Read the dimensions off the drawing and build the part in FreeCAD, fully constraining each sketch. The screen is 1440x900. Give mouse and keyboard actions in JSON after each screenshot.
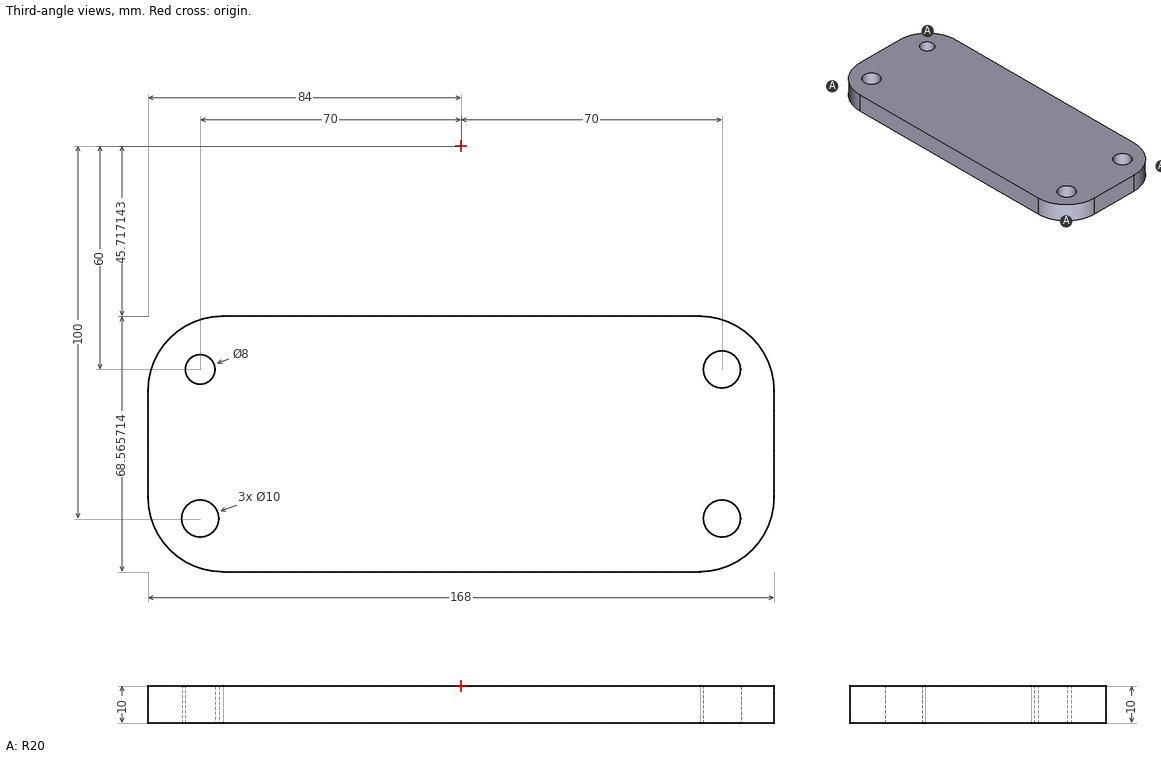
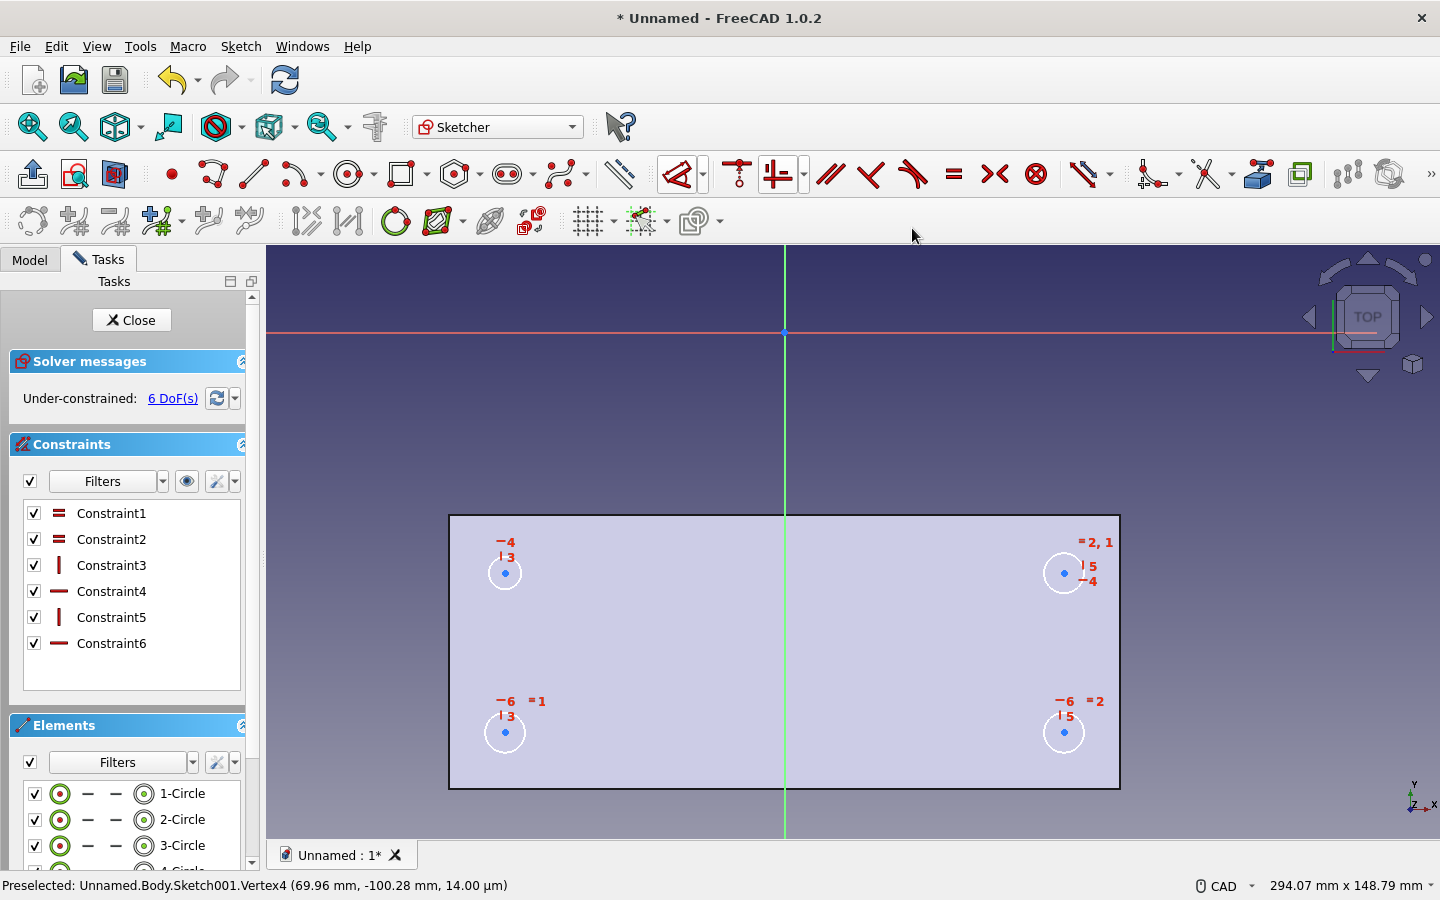
{"action": "scroll", "coordinate": [516, 562], "scroll_direction": "up", "scroll_amount": 2}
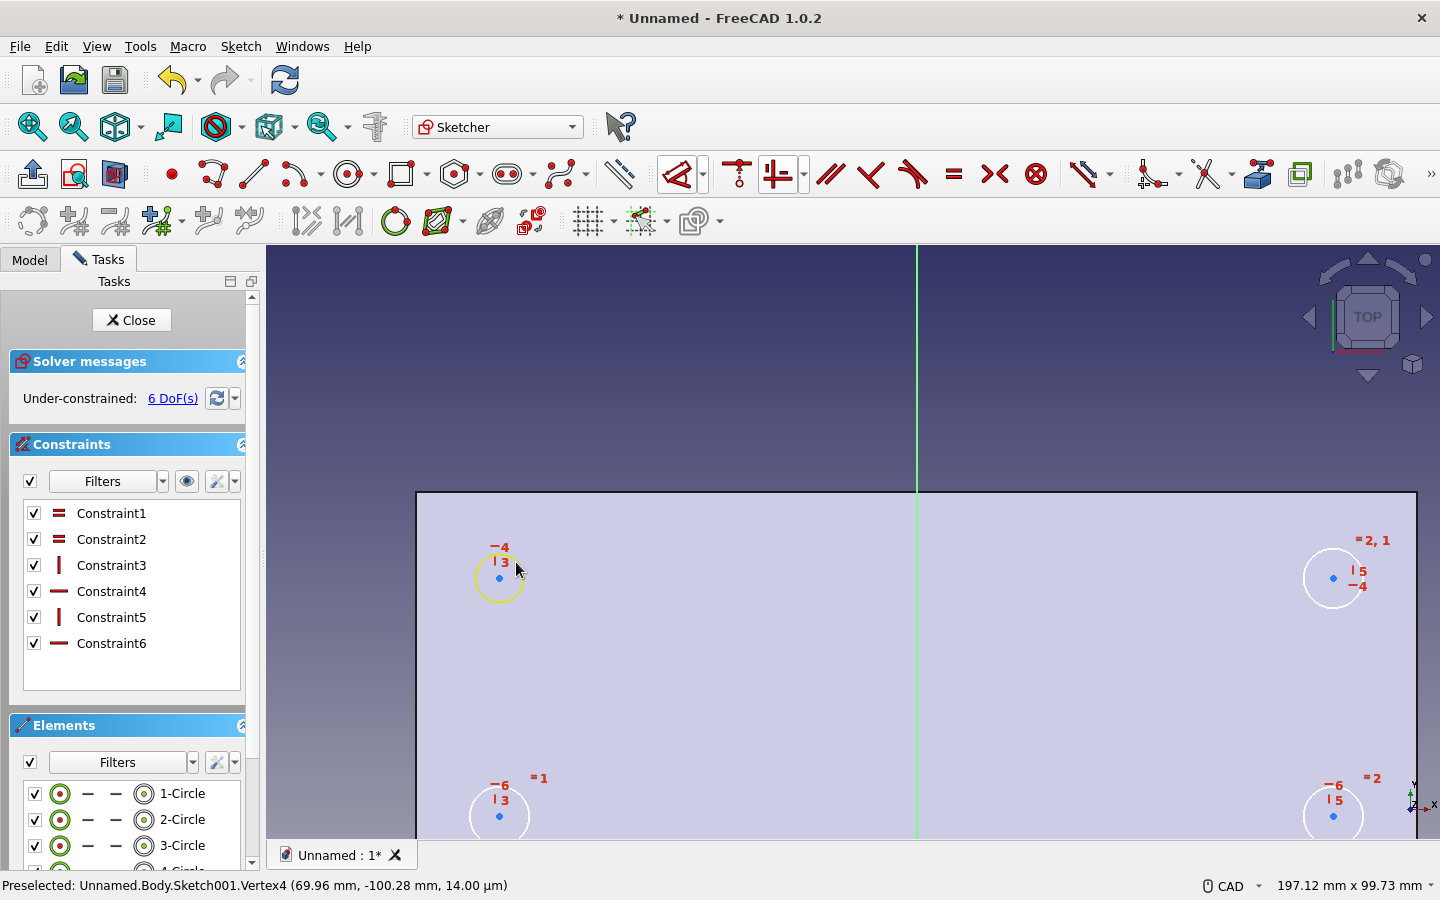
{"action": "left_click", "coordinate": [517, 561]}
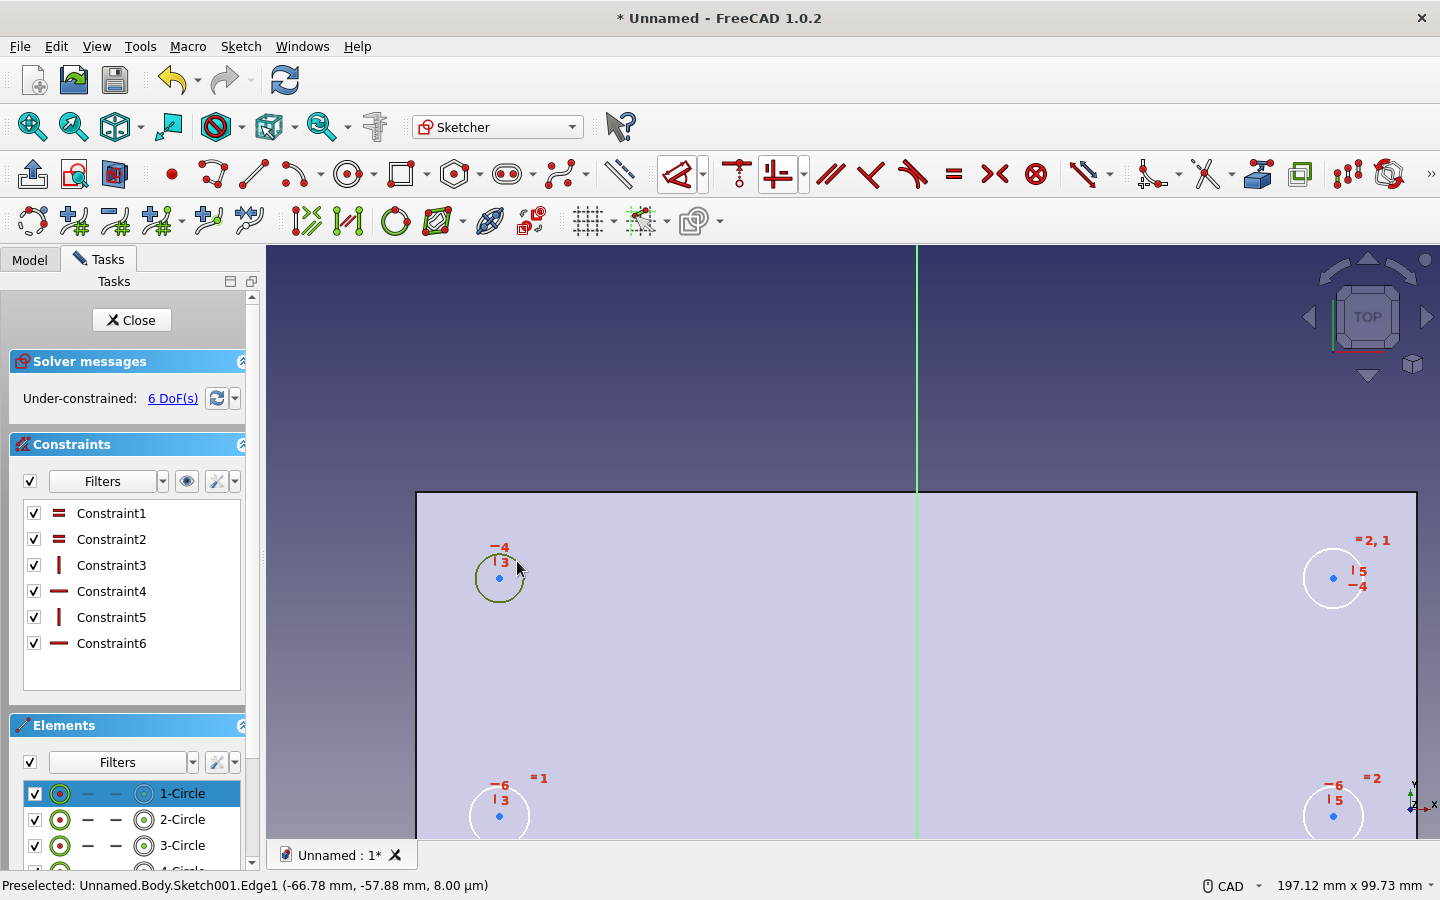
{"action": "left_click", "coordinate": [702, 174]}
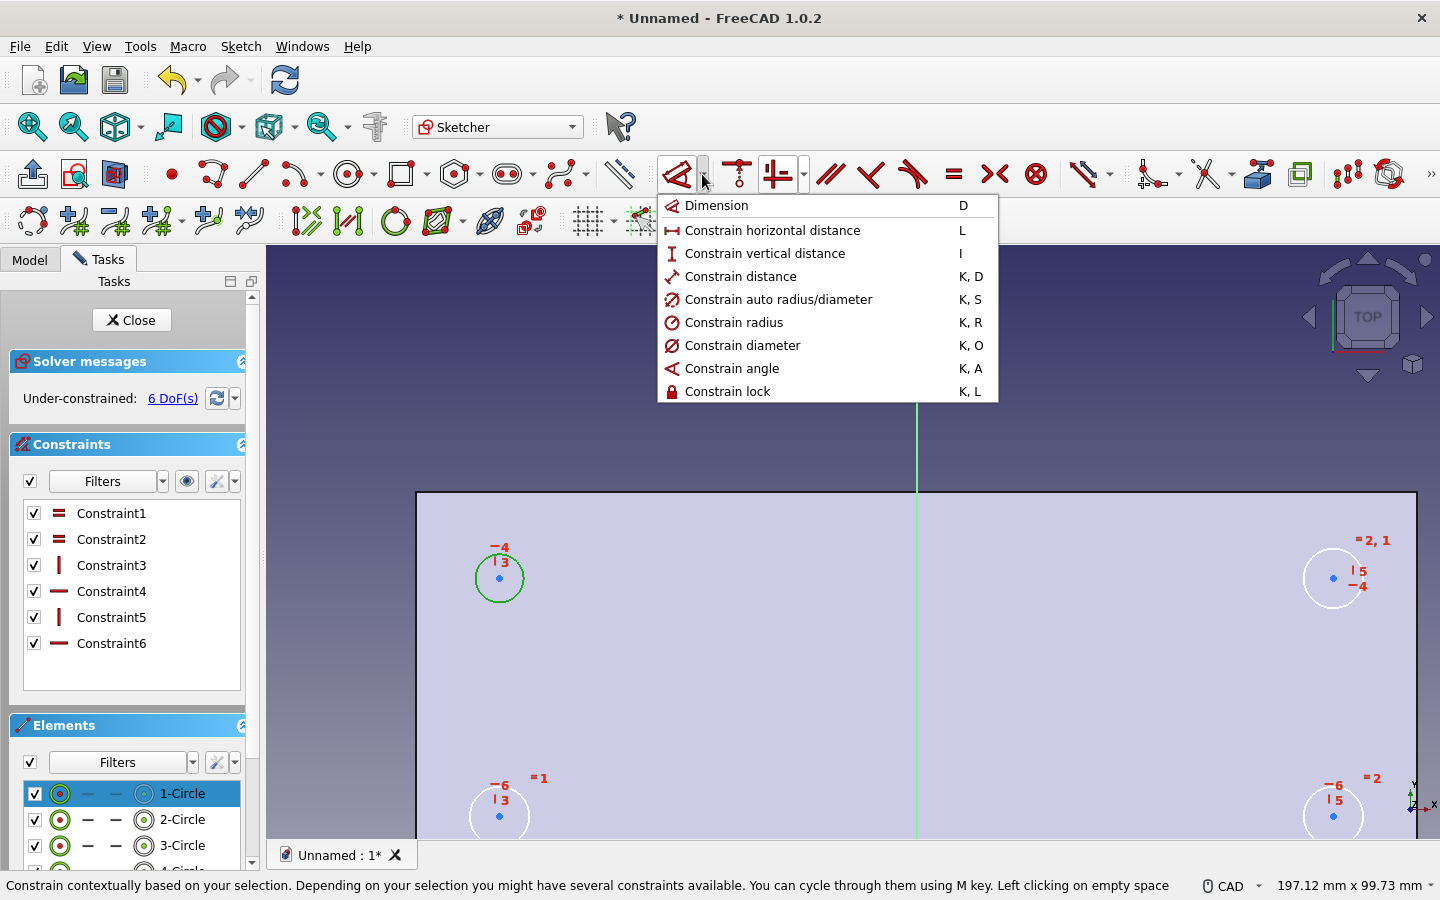
{"action": "left_click", "coordinate": [828, 346]}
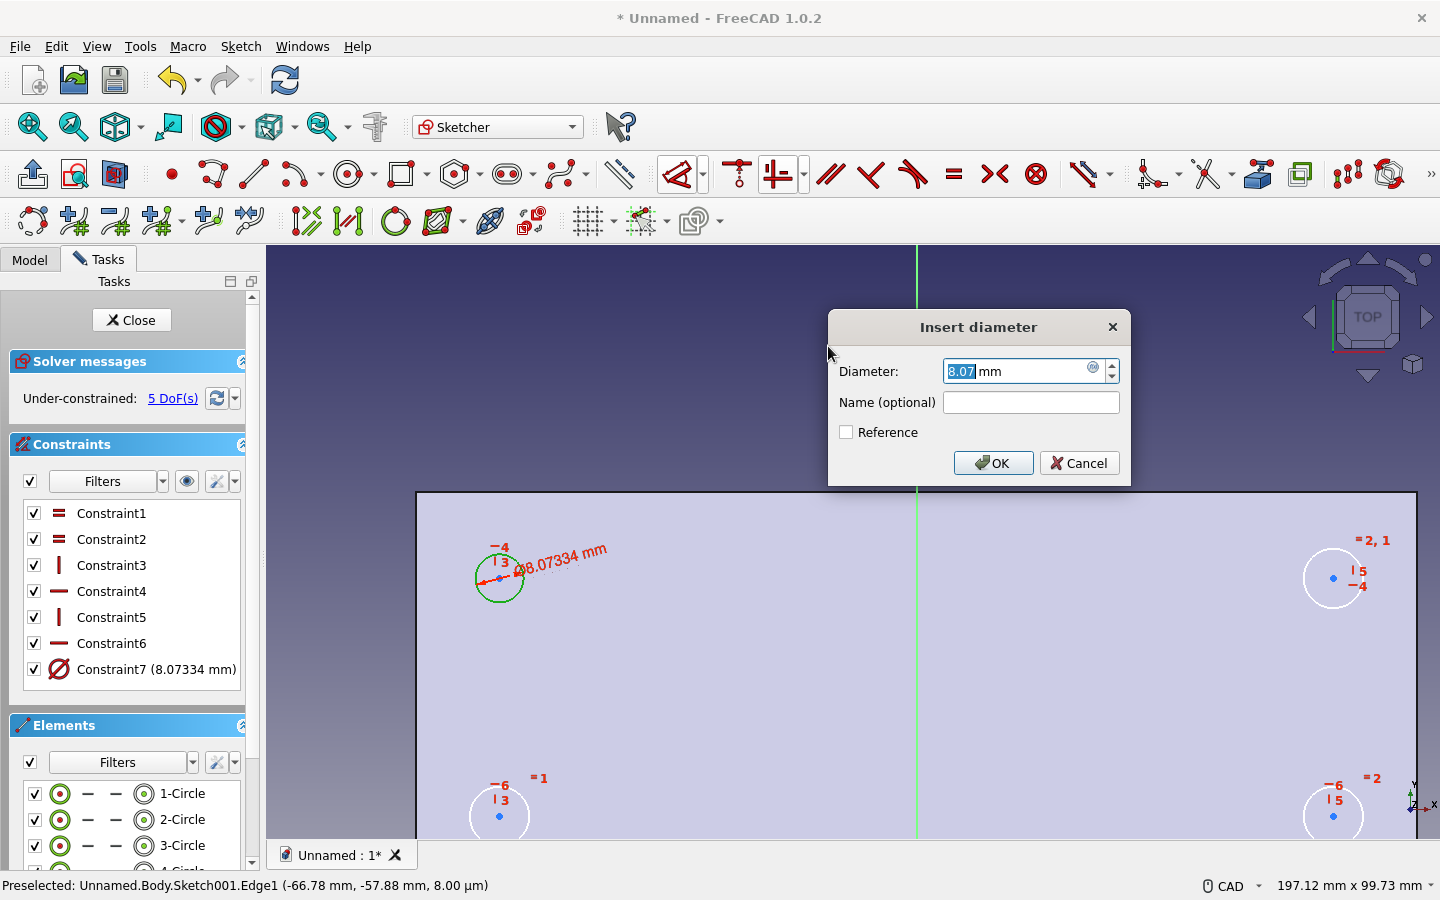
{"action": "type", "text": "8"}
{"action": "key", "text": "Return"}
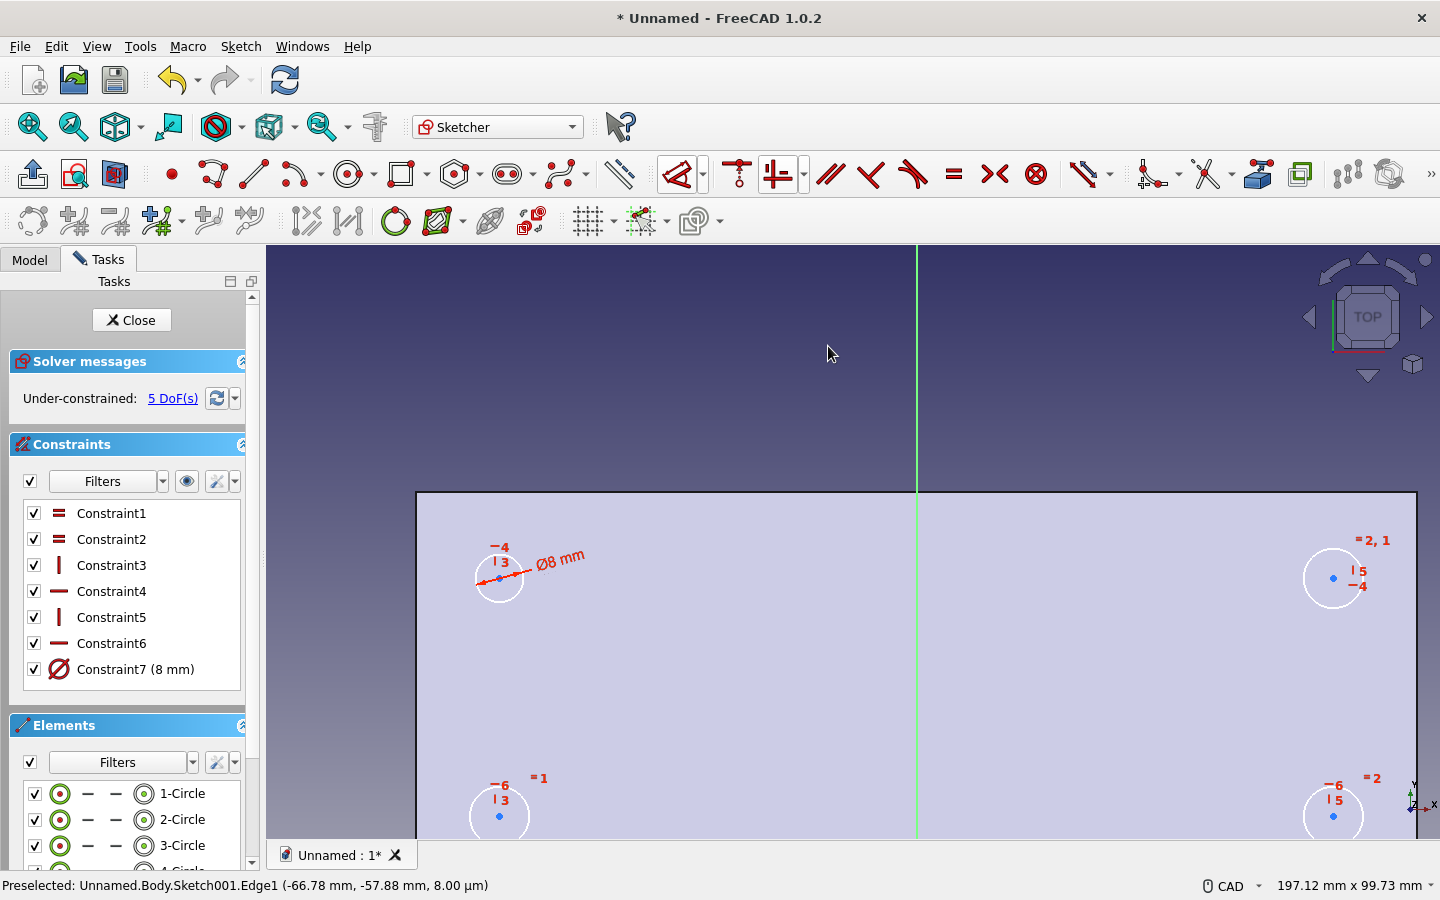
{"action": "left_click", "coordinate": [521, 795]}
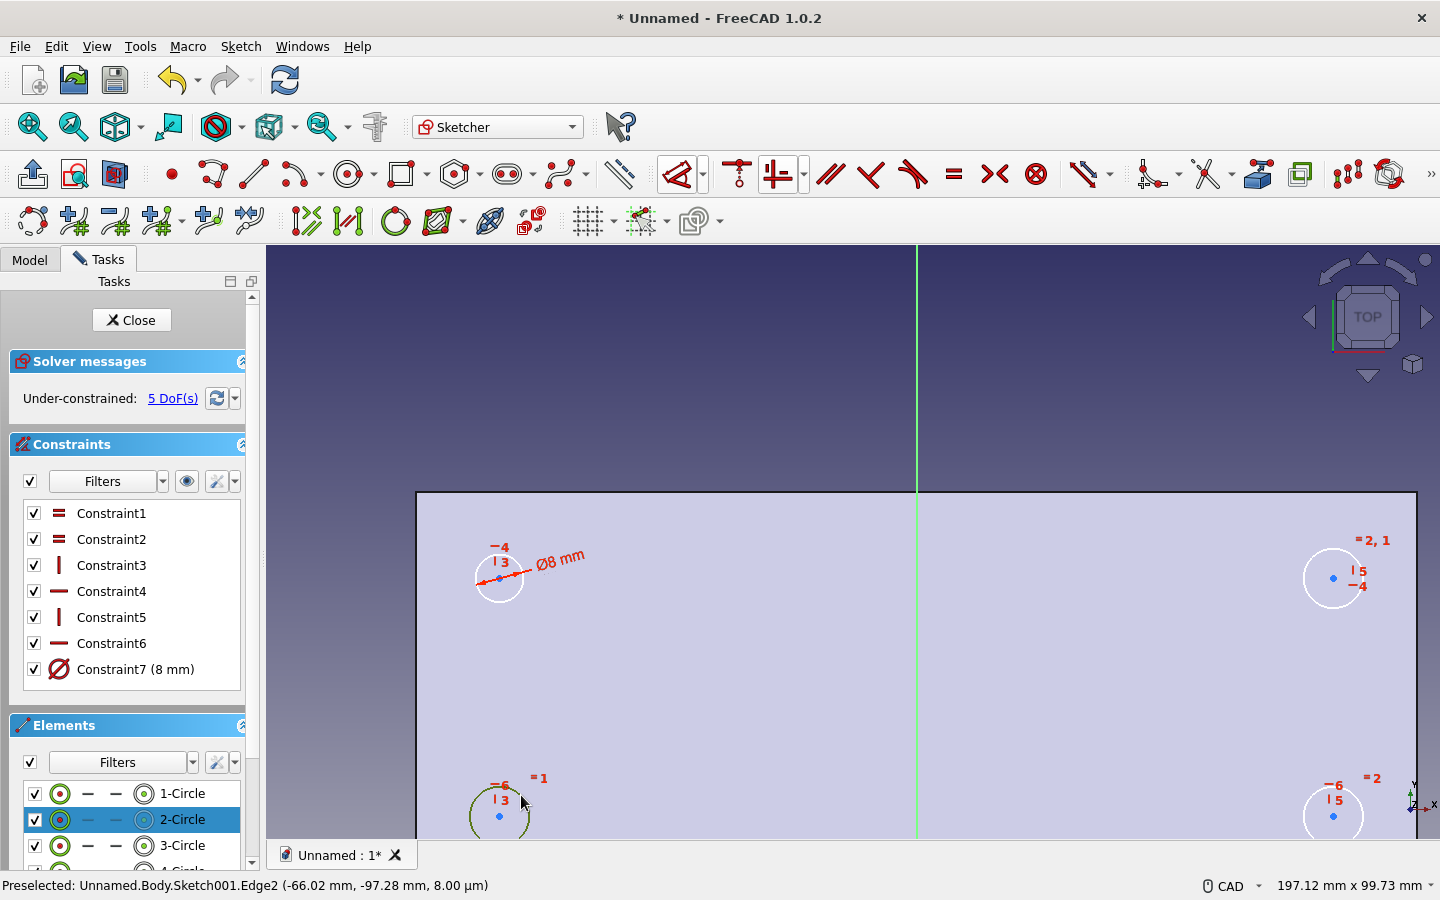
{"action": "left_click", "coordinate": [702, 174]}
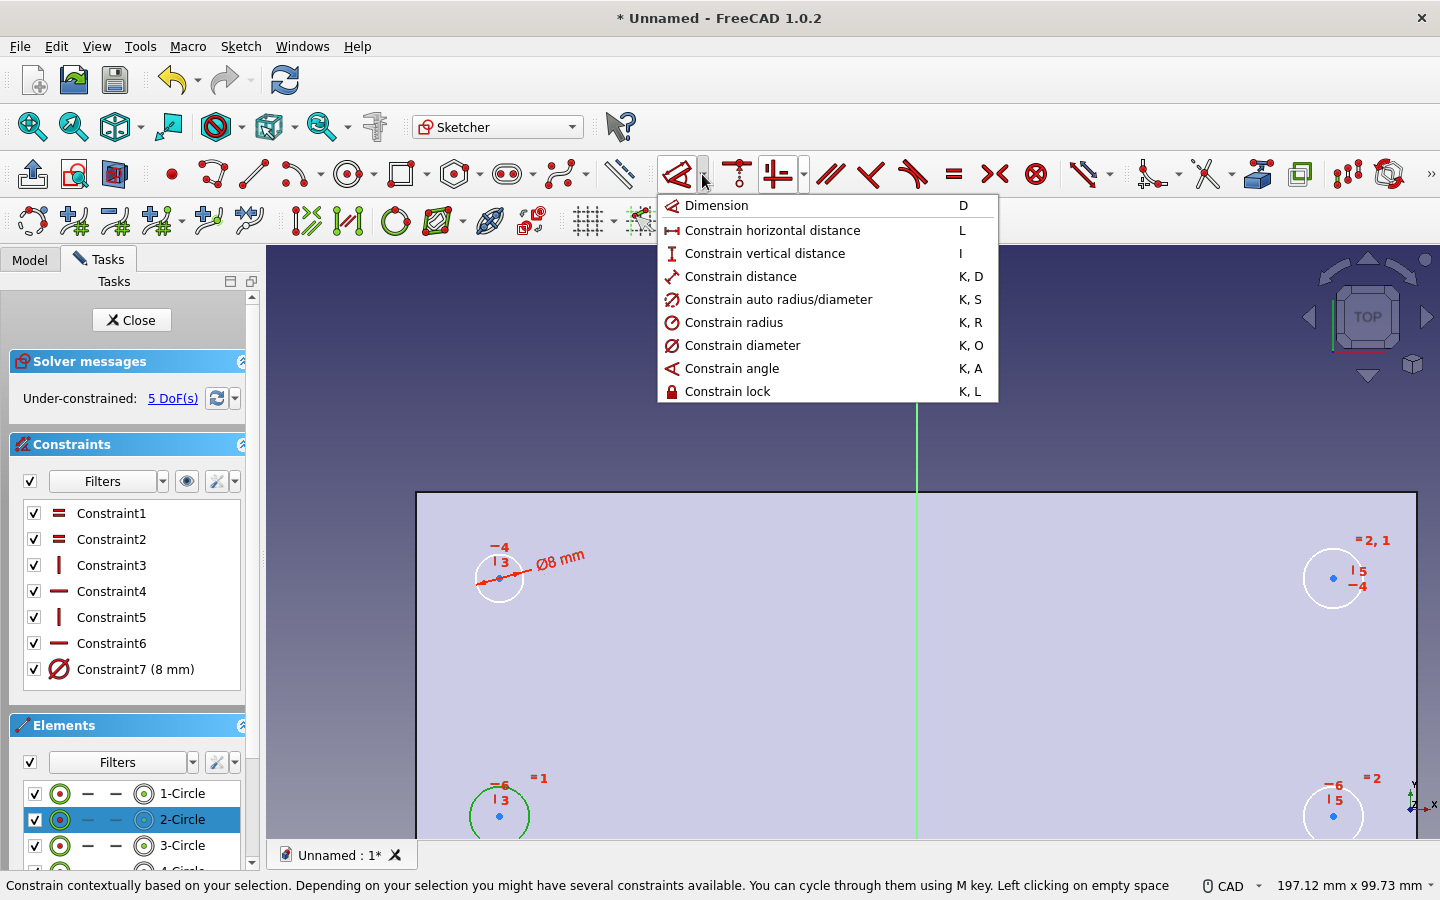
{"action": "left_click", "coordinate": [828, 346]}